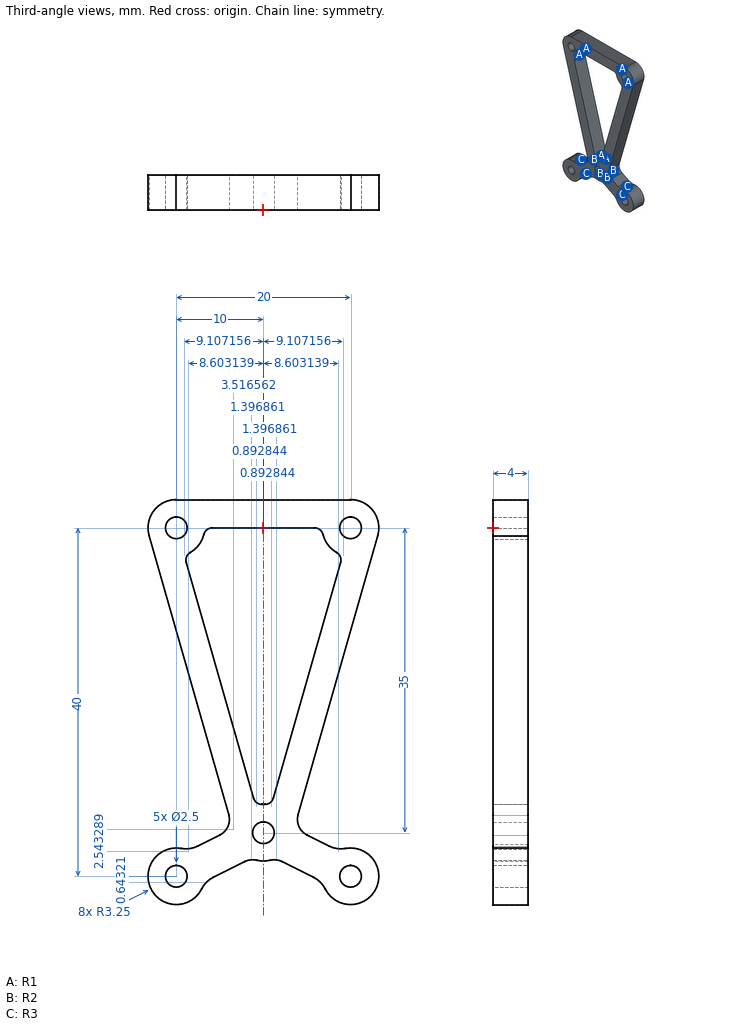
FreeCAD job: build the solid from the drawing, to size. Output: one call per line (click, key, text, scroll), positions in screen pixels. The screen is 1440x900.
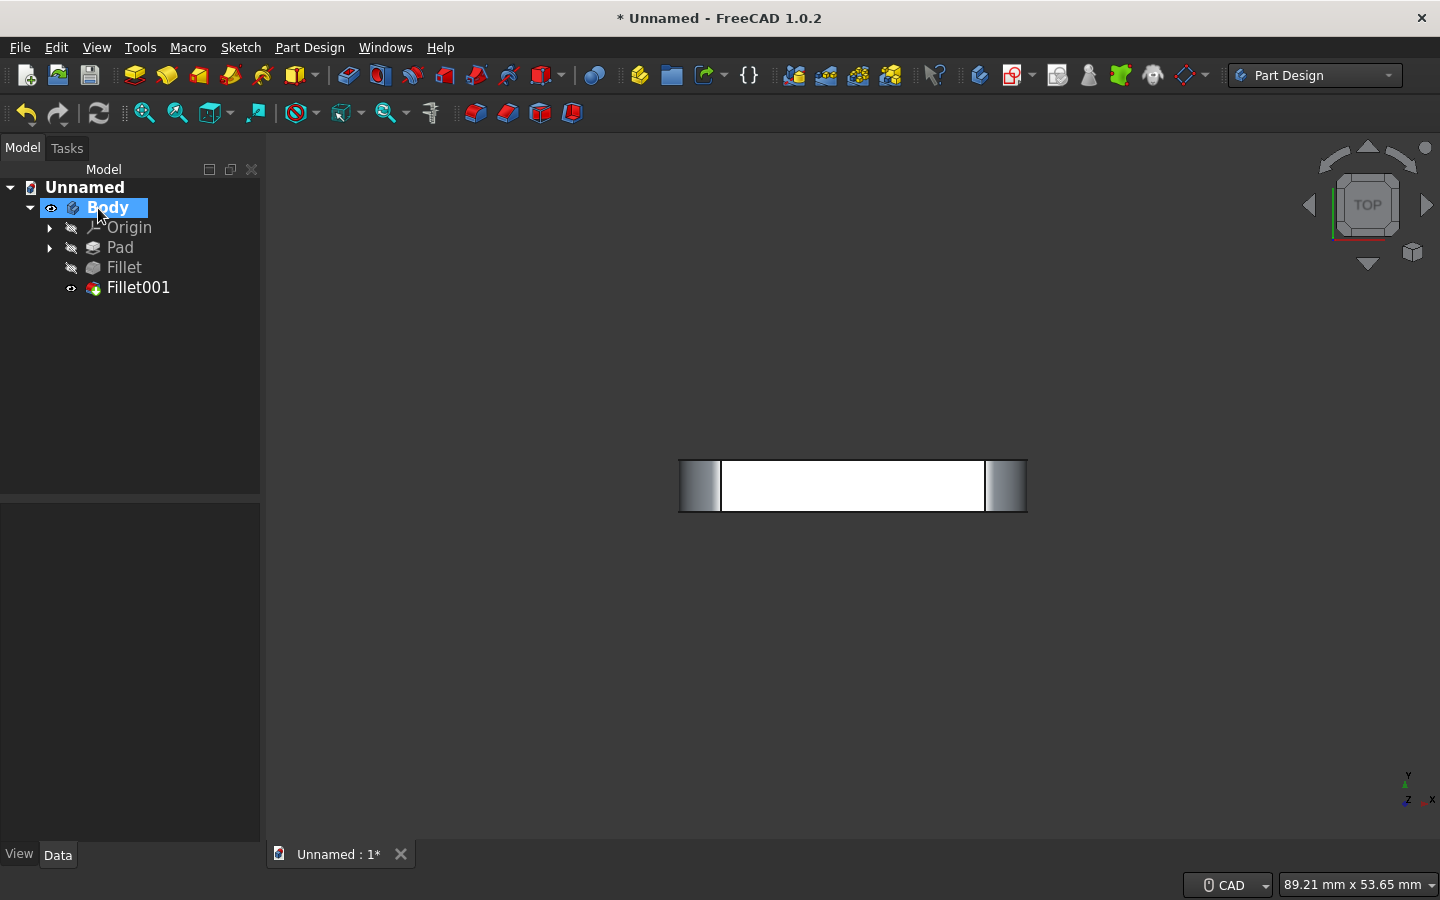
click(146, 114)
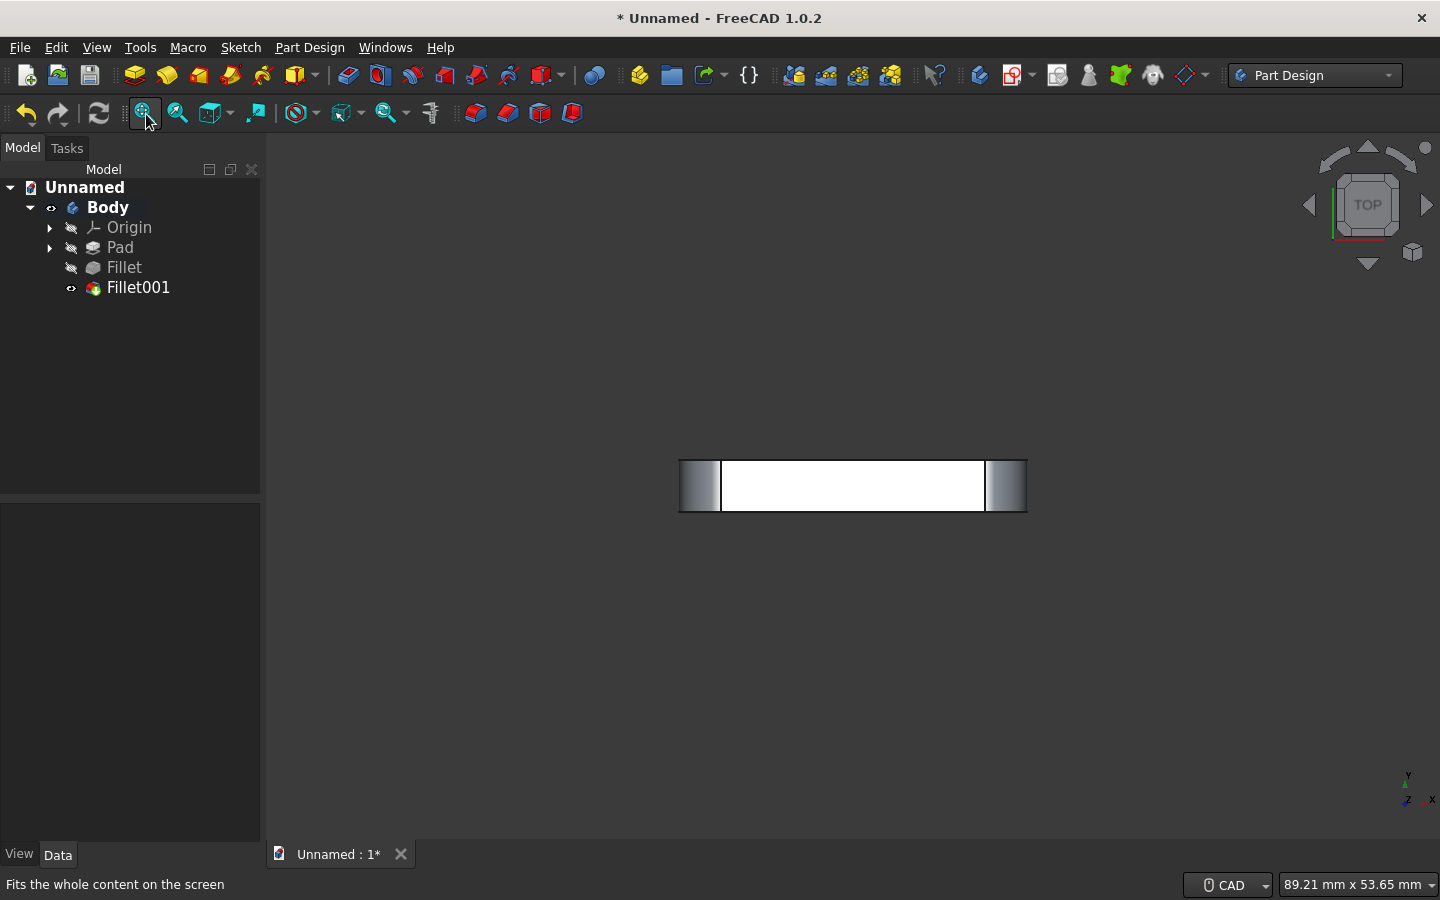
key(0)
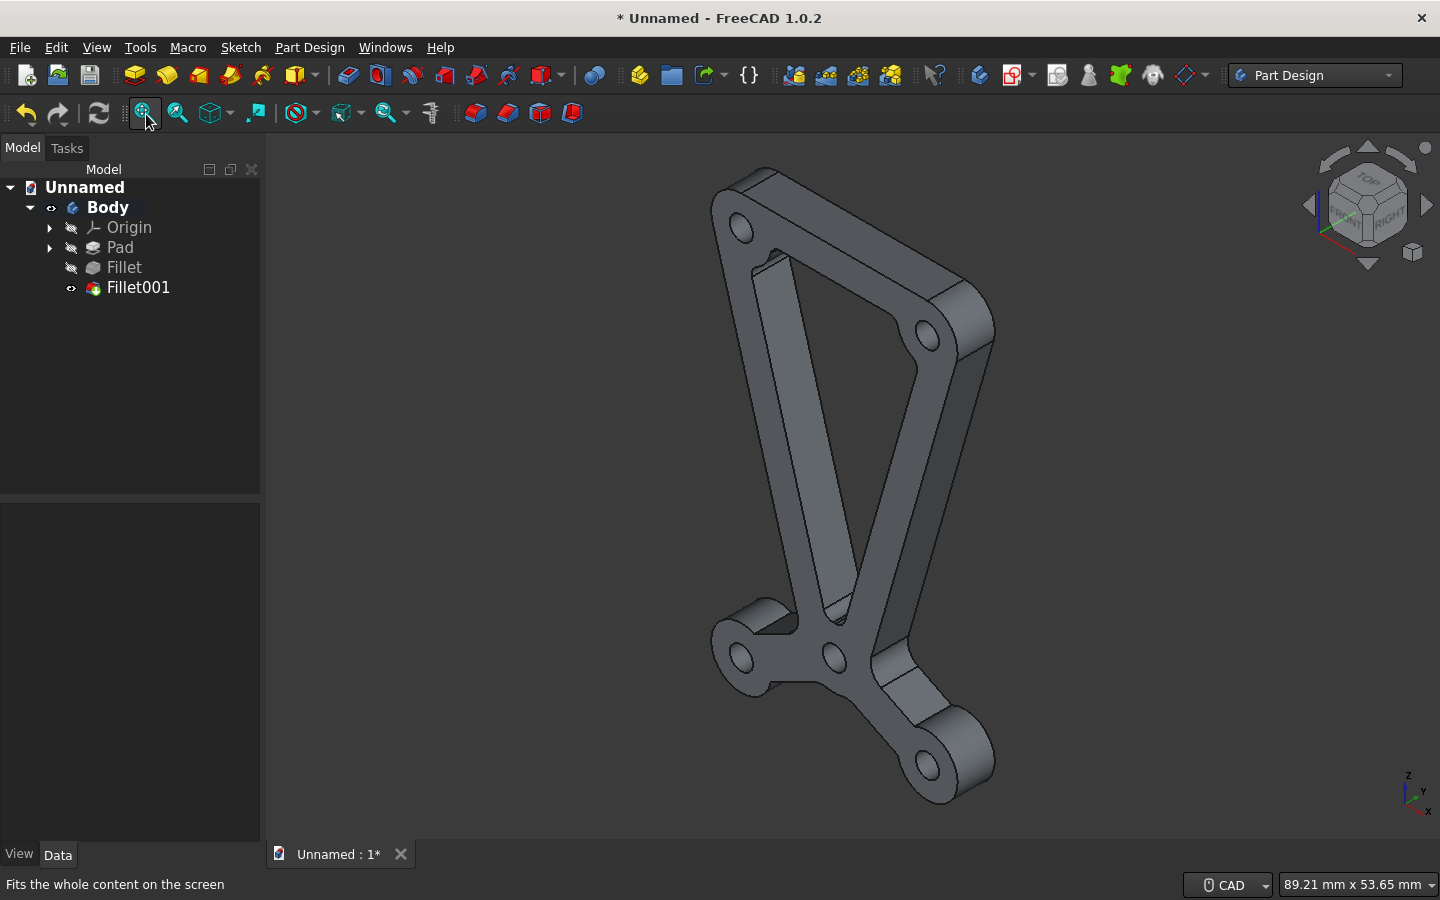
key(1)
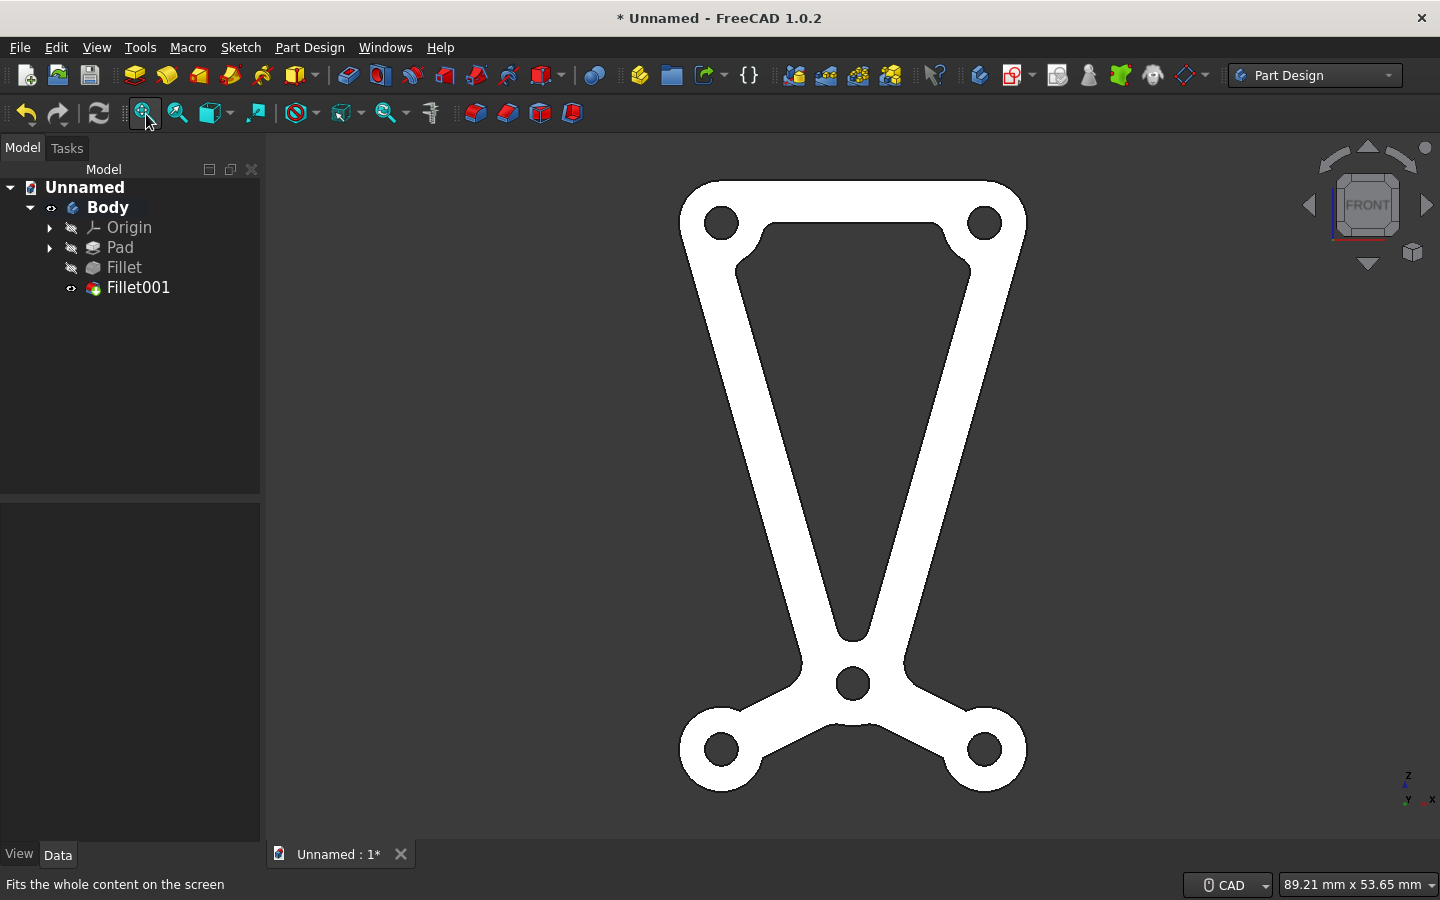
key(3)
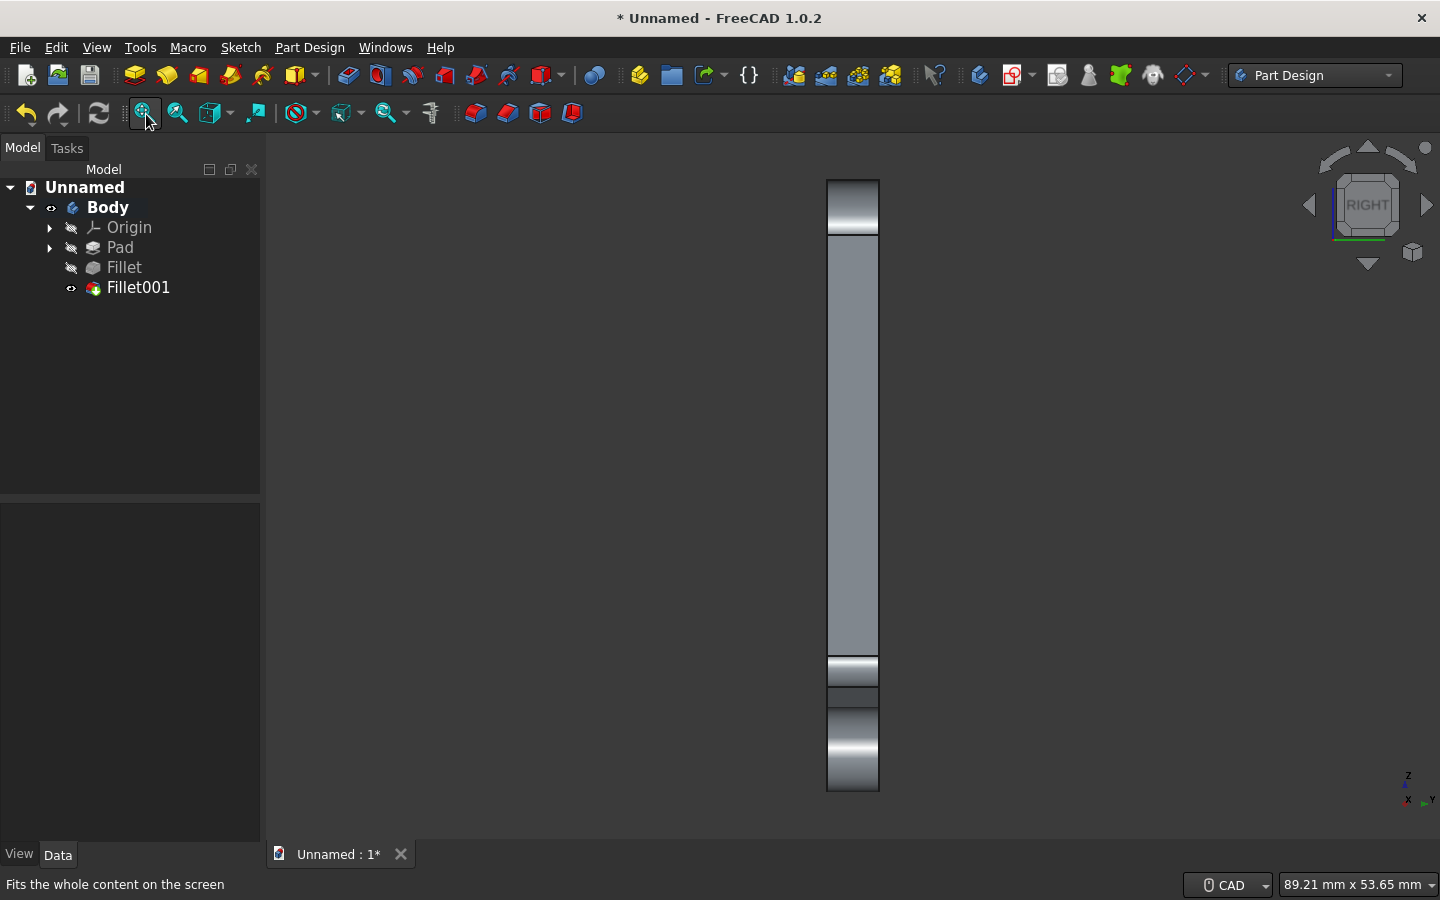
key(5)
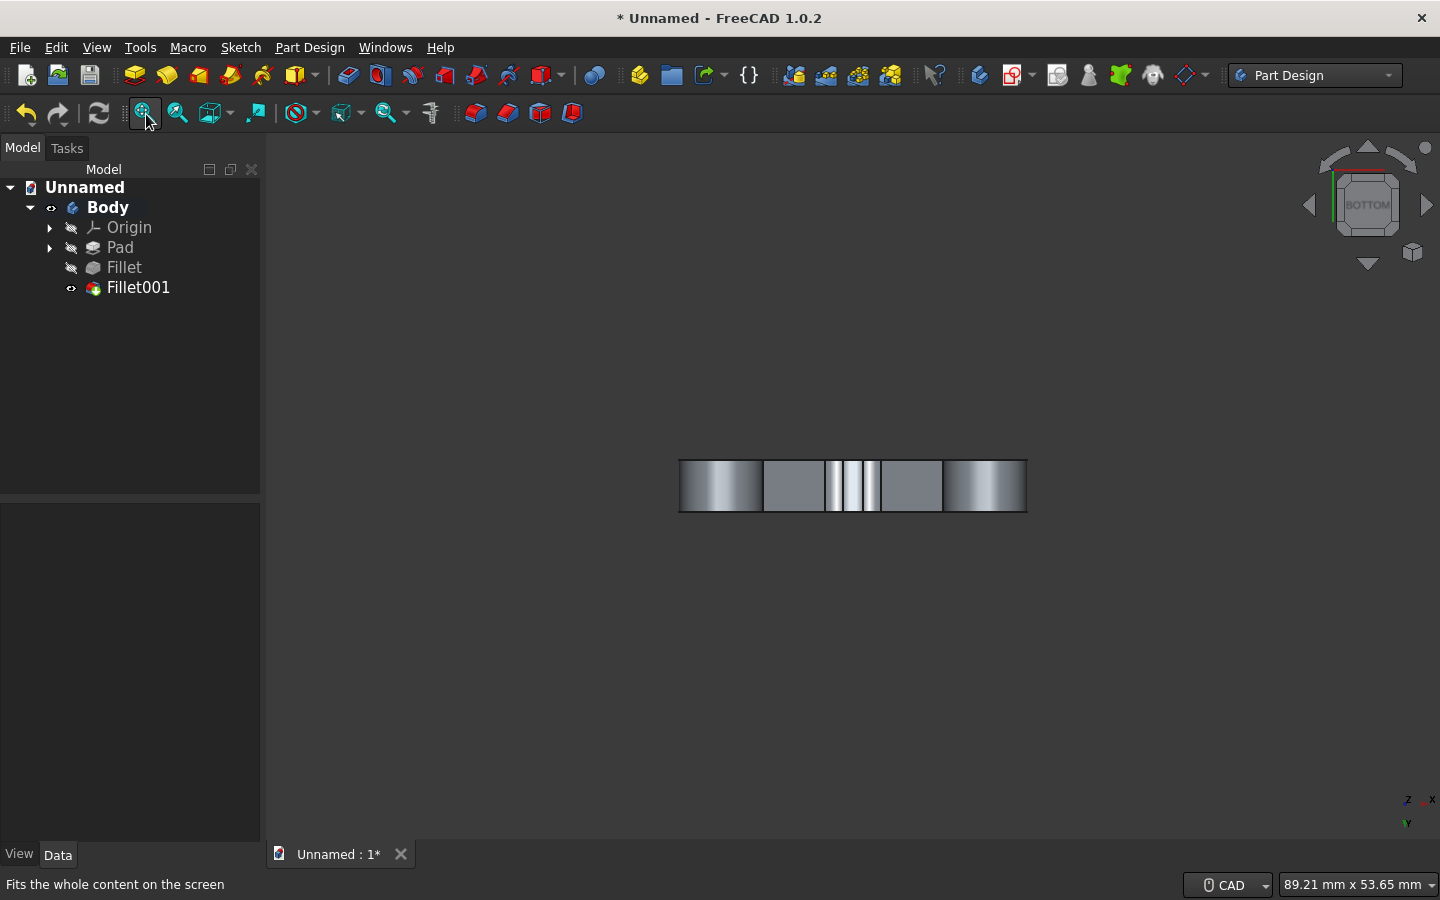
click(146, 114)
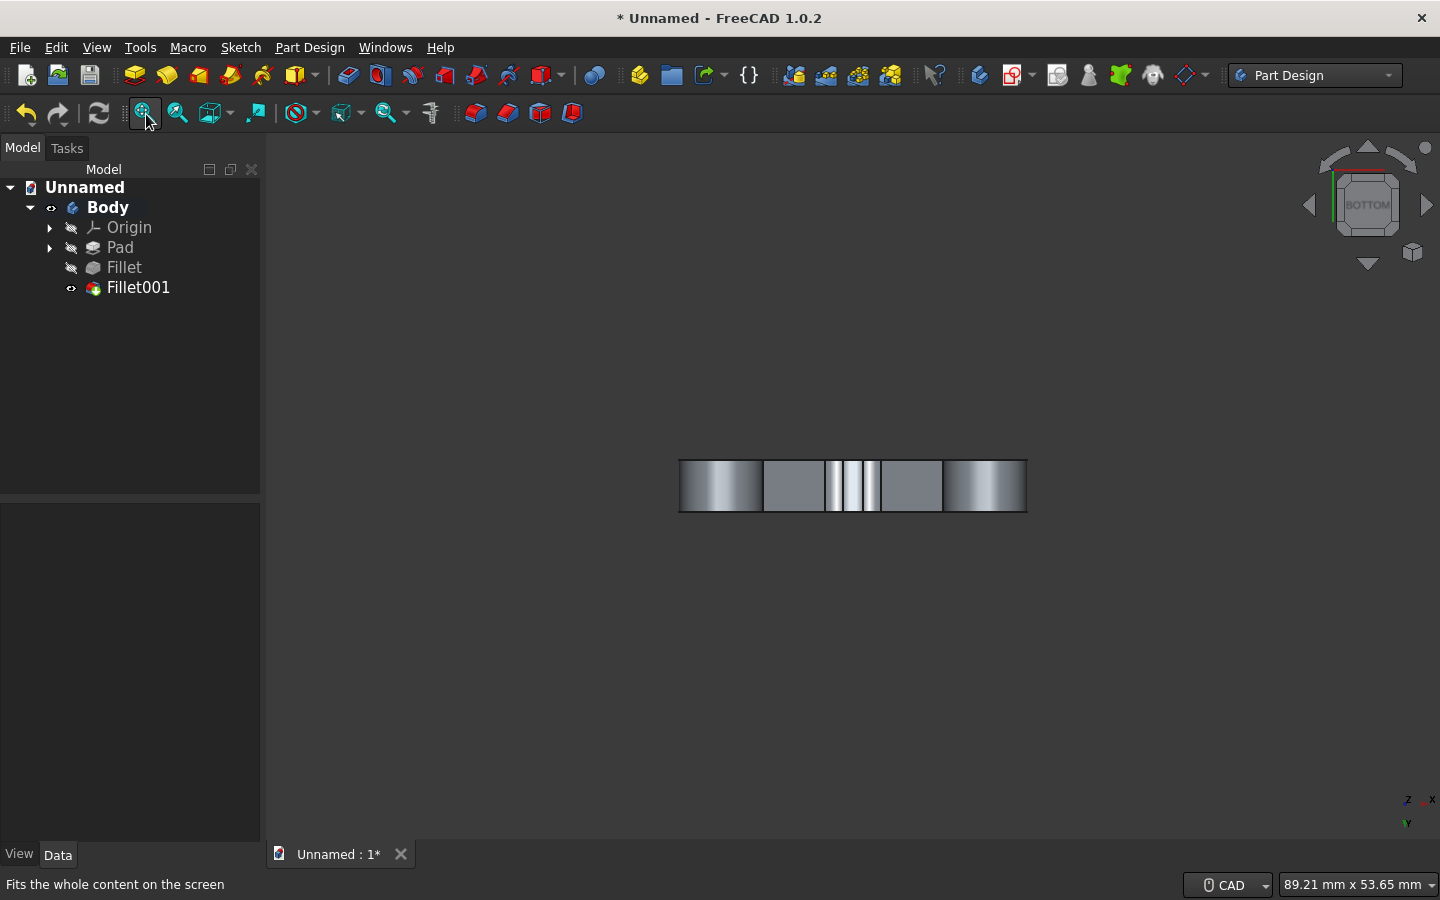
key(4)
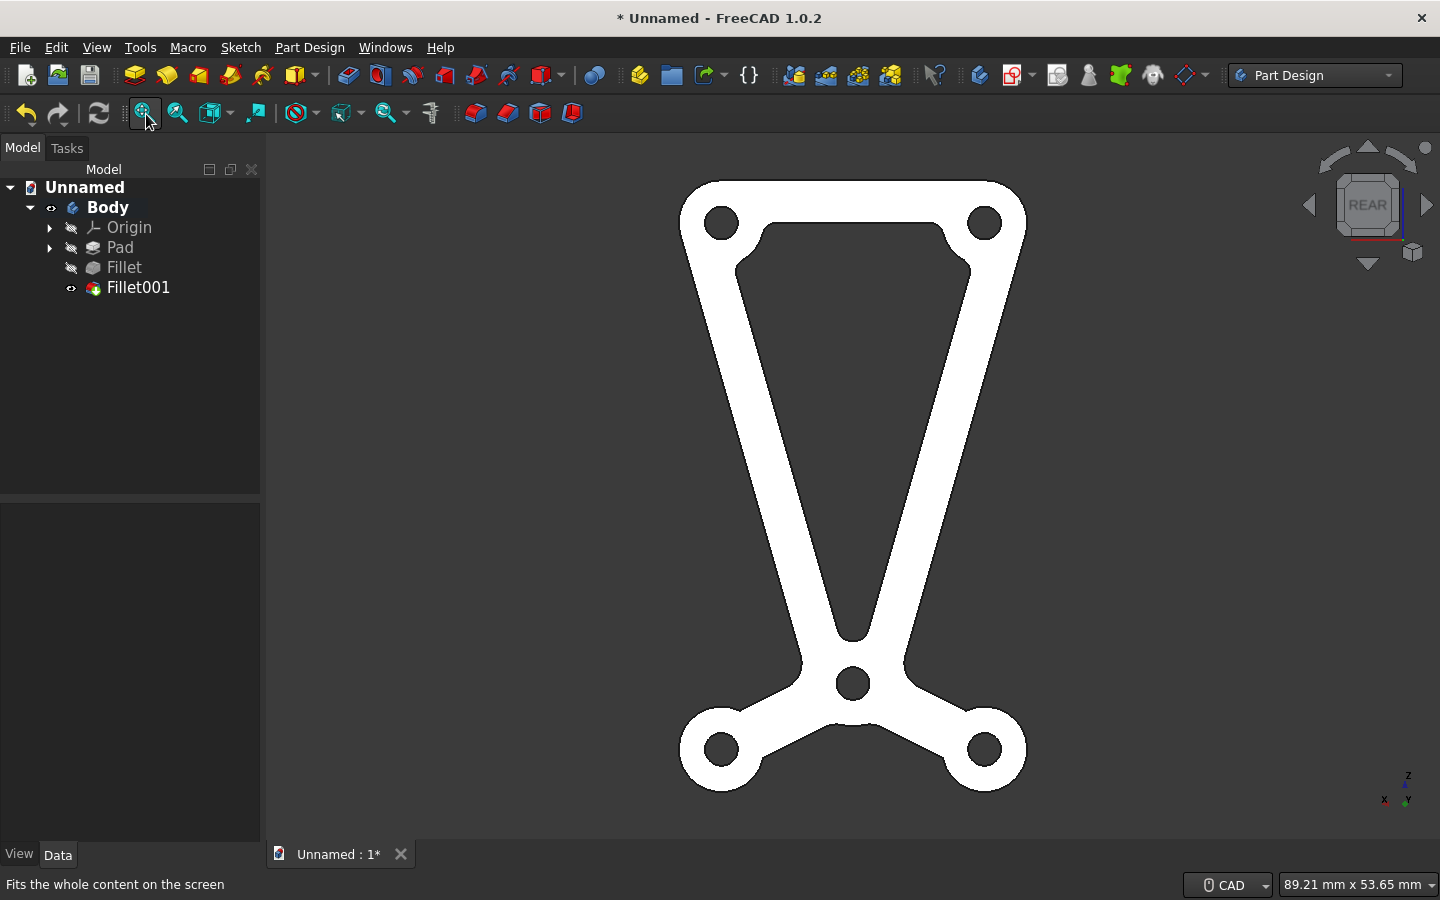
key(6)